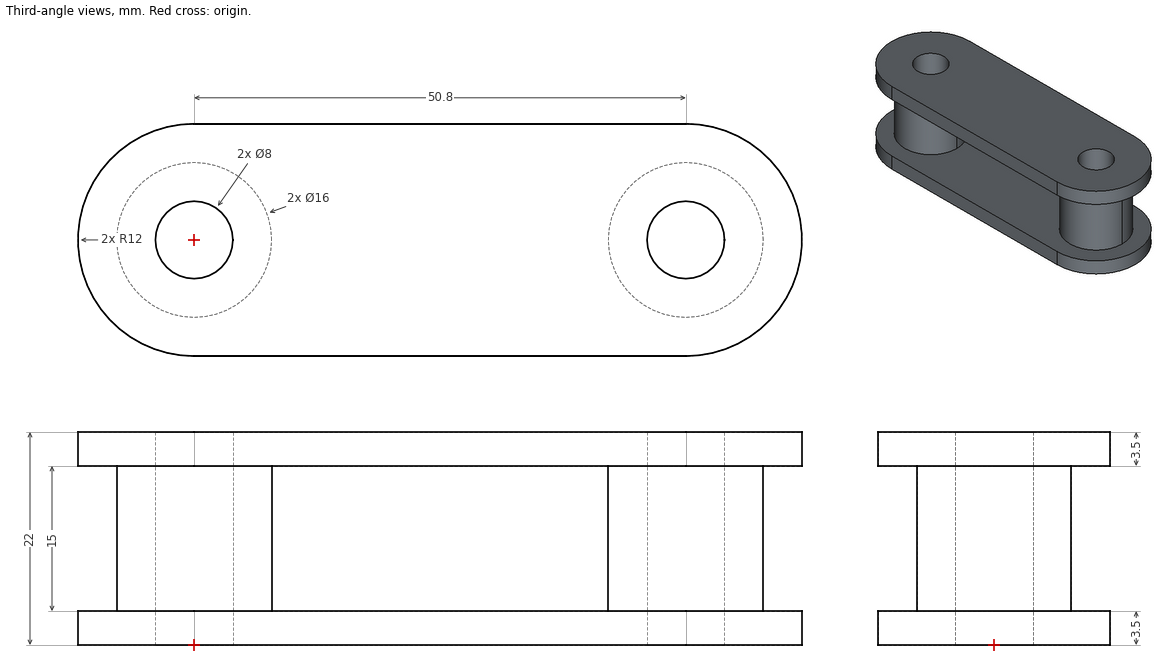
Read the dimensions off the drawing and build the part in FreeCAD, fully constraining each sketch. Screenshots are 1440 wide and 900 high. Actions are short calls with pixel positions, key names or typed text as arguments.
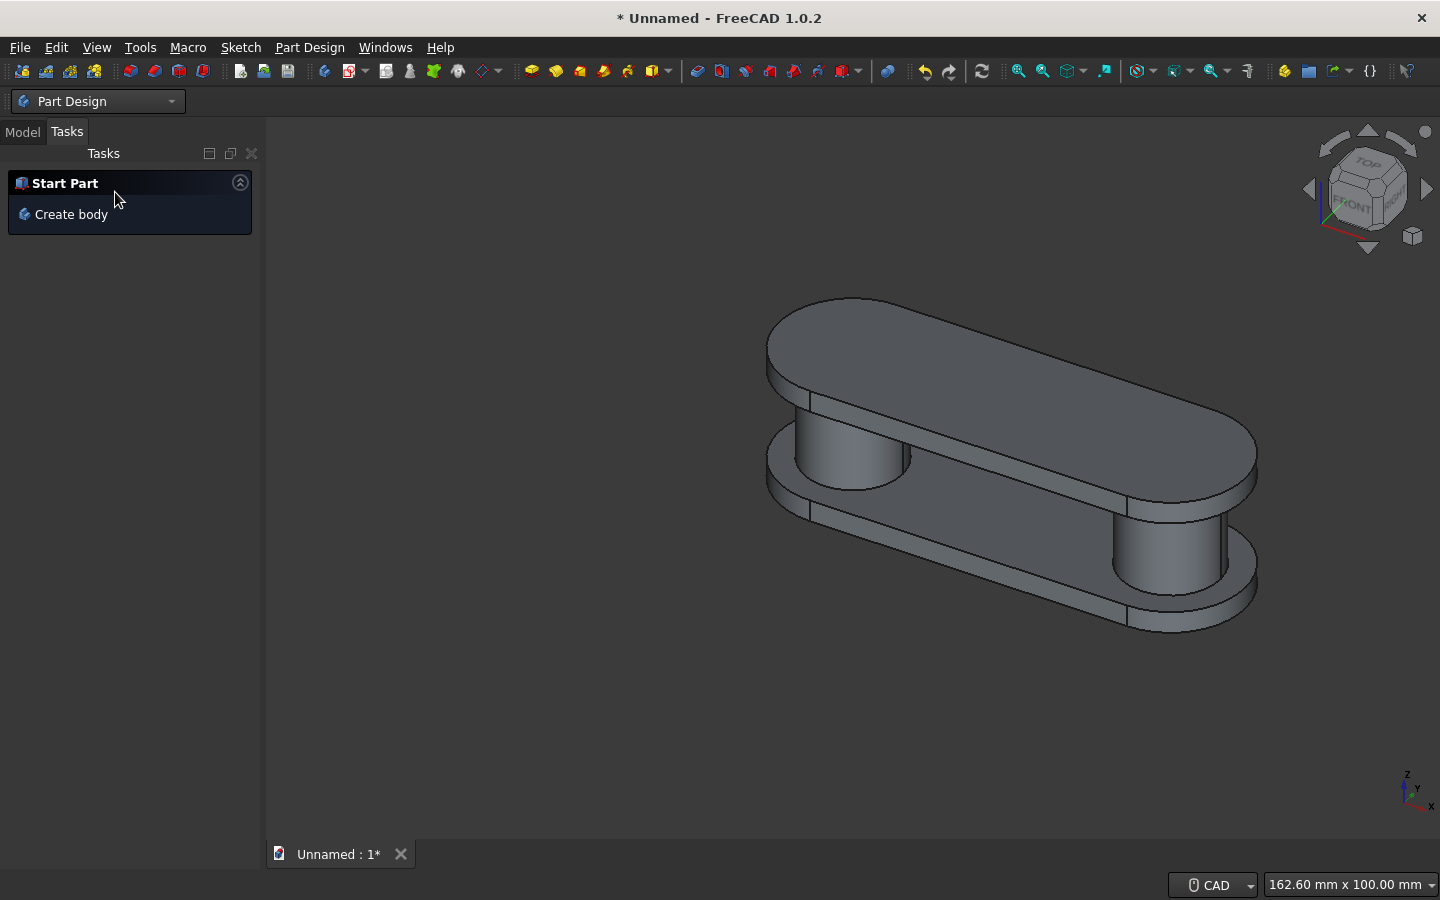
click(1145, 444)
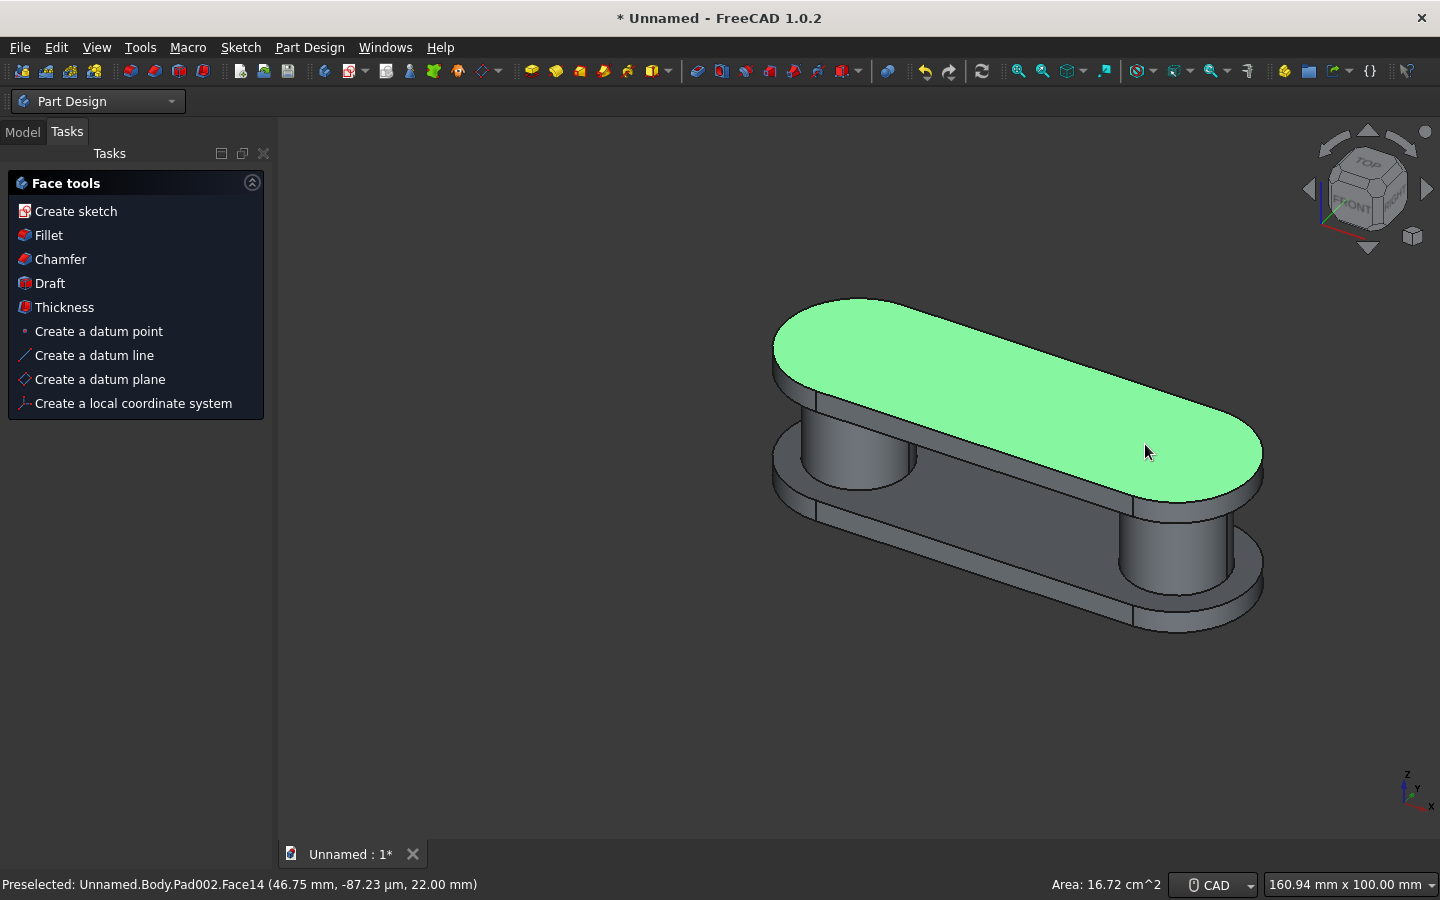
click(350, 72)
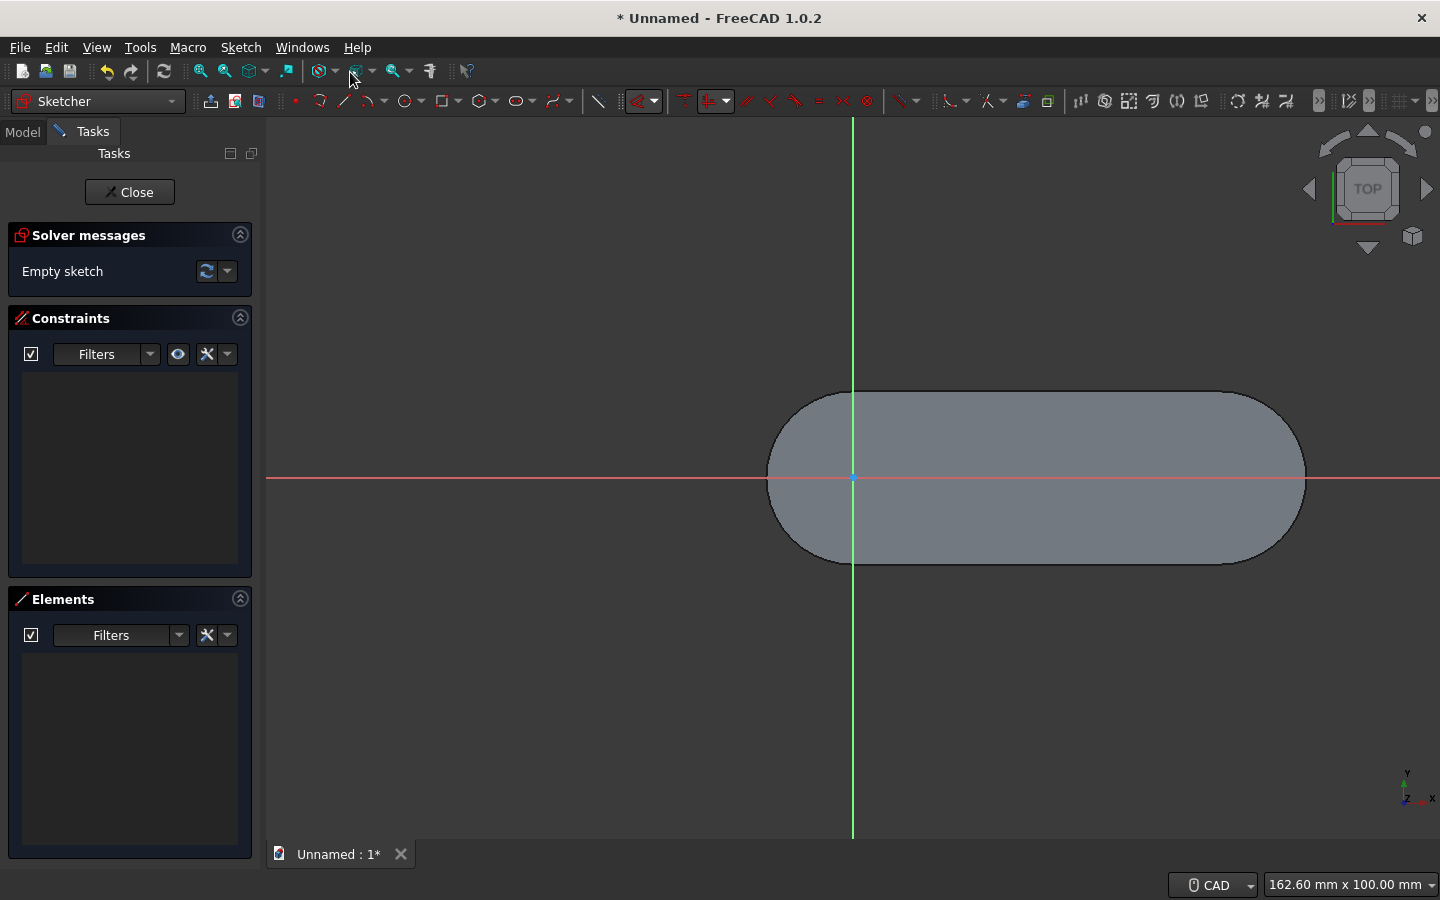
scroll(1275, 478, up, 2)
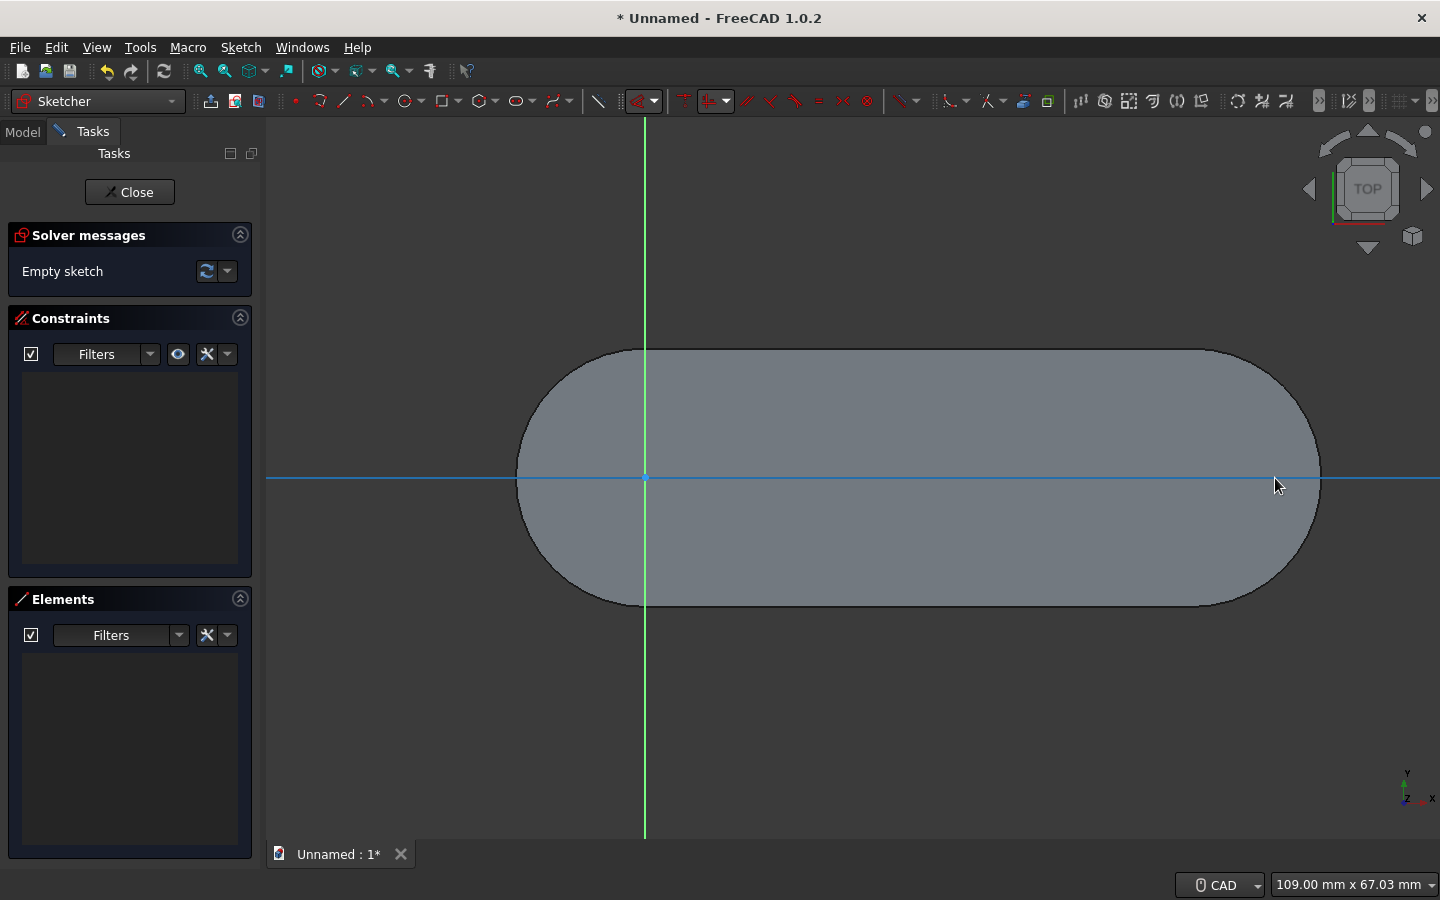
click(406, 102)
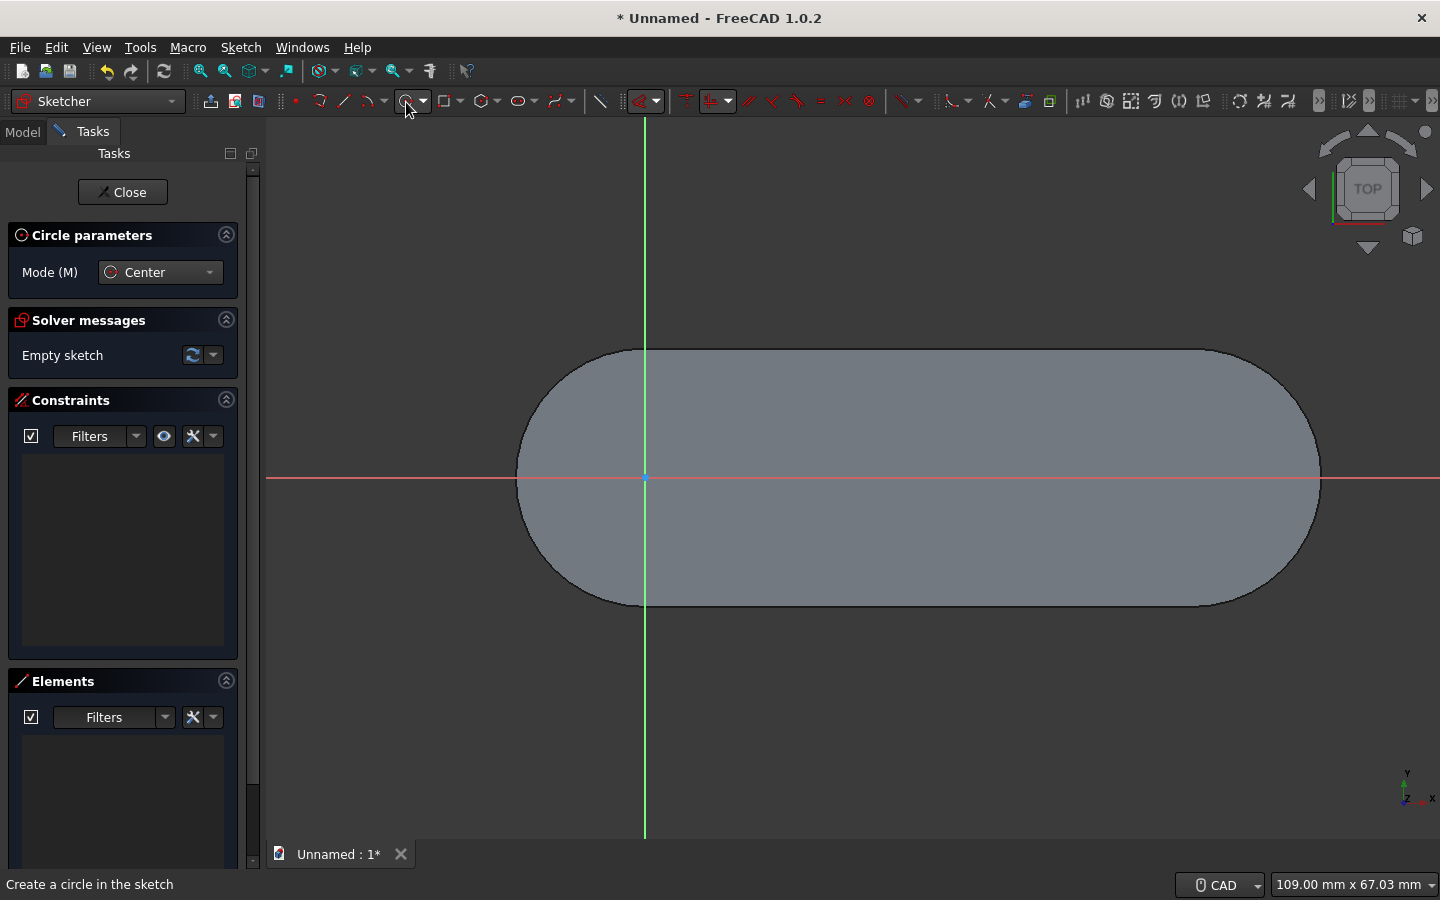
click(645, 478)
move(675, 447)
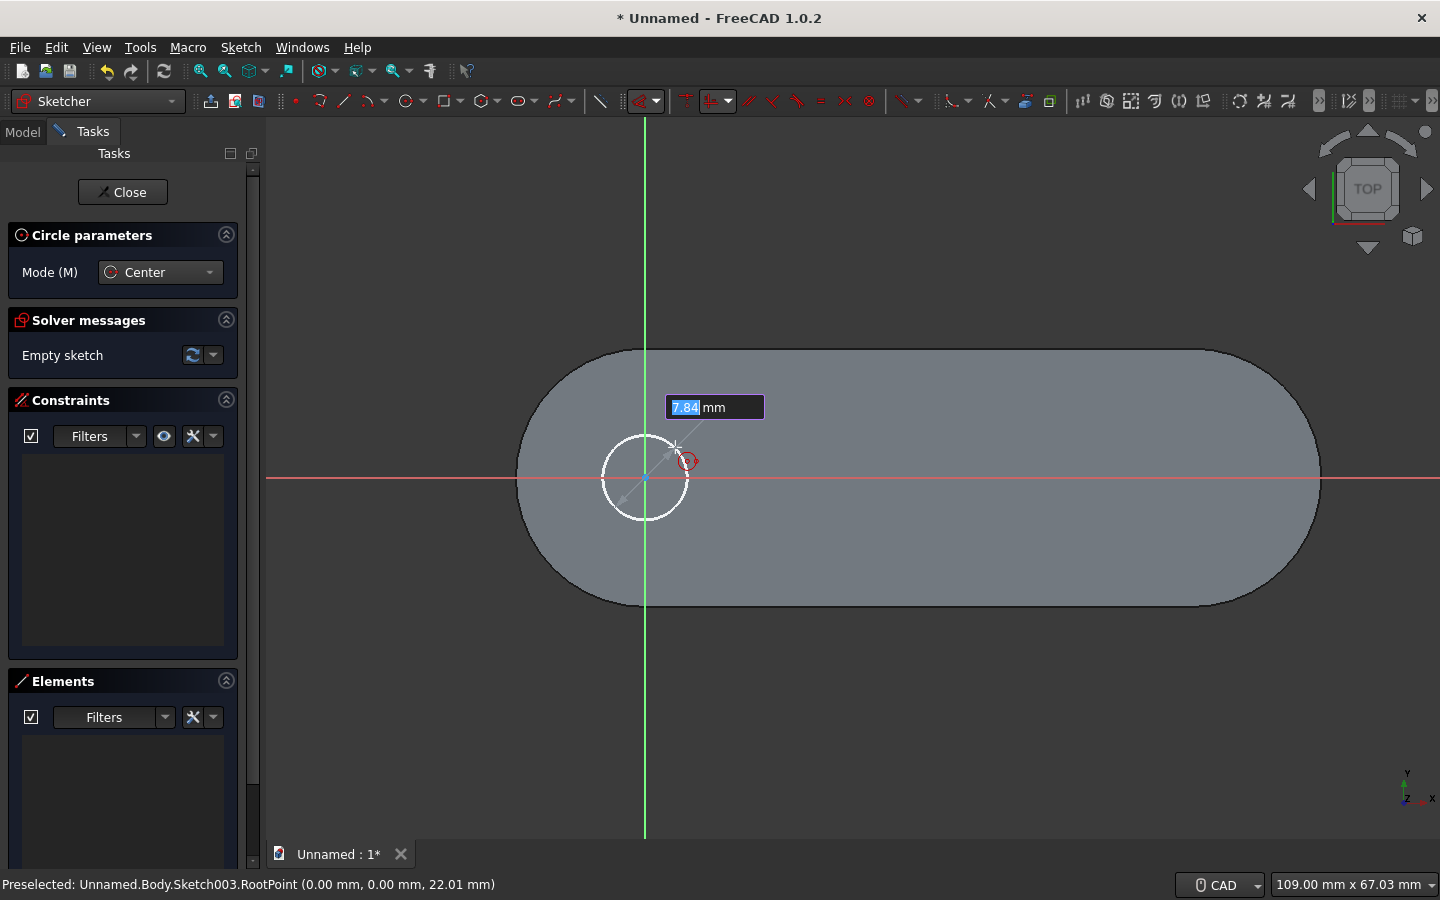
text(8)
key(Return)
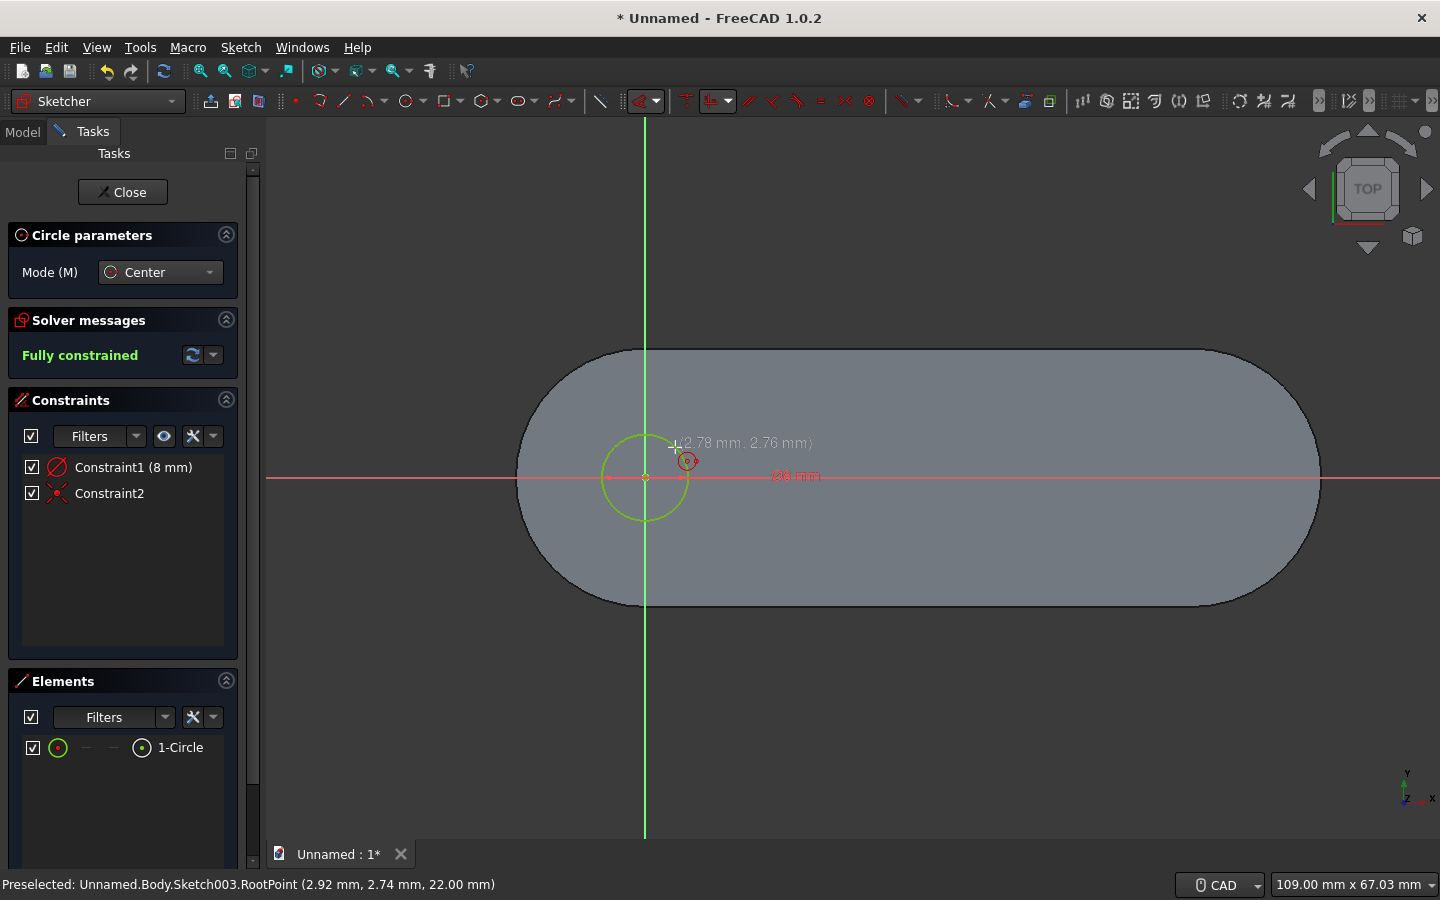
click(1192, 478)
move(1223, 447)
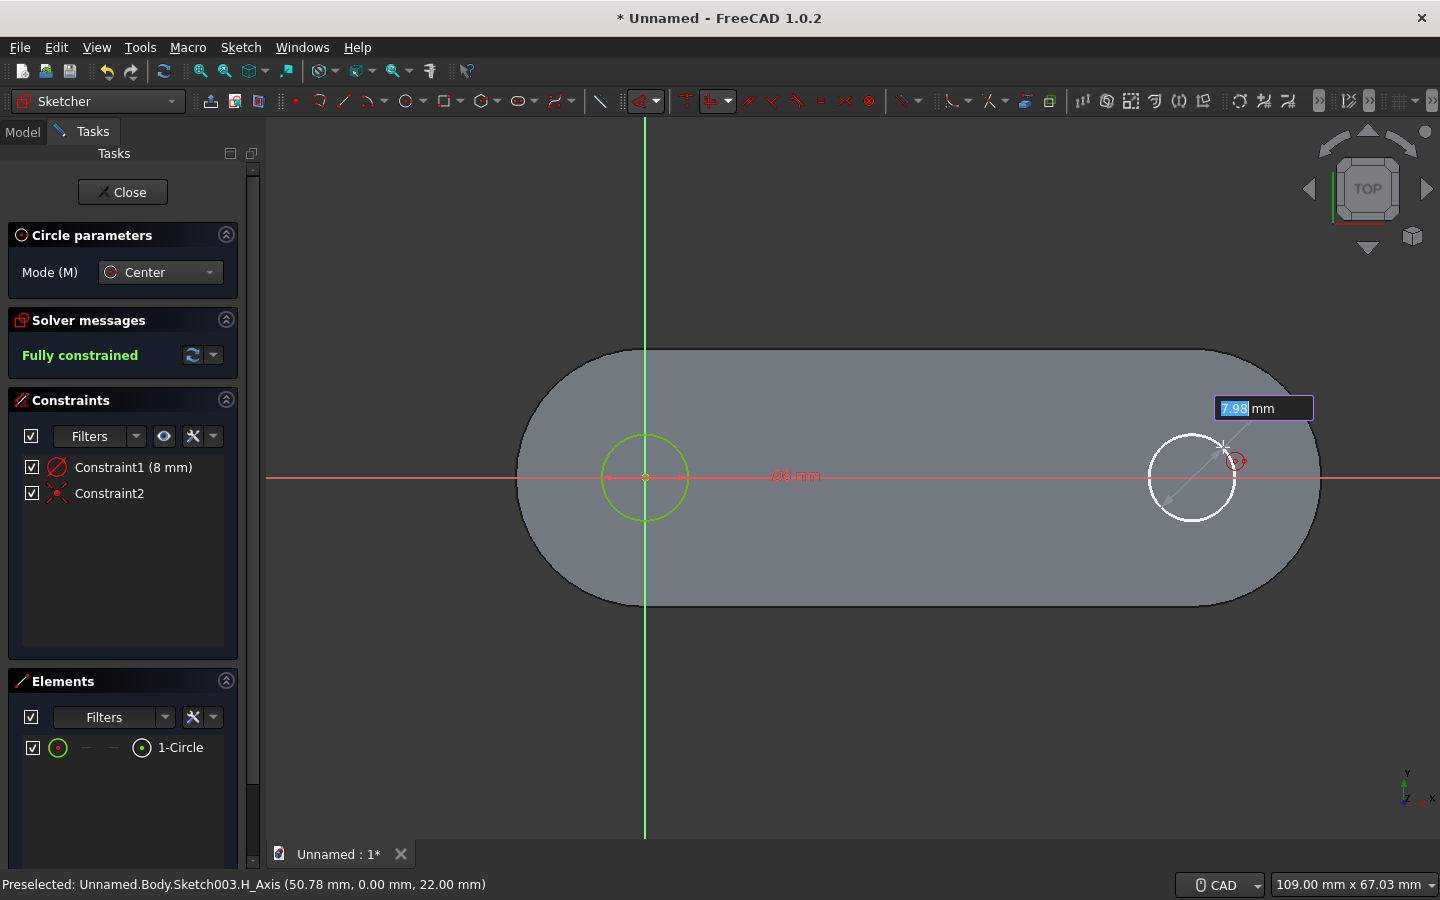
text(8)
key(Return)
key(Escape)